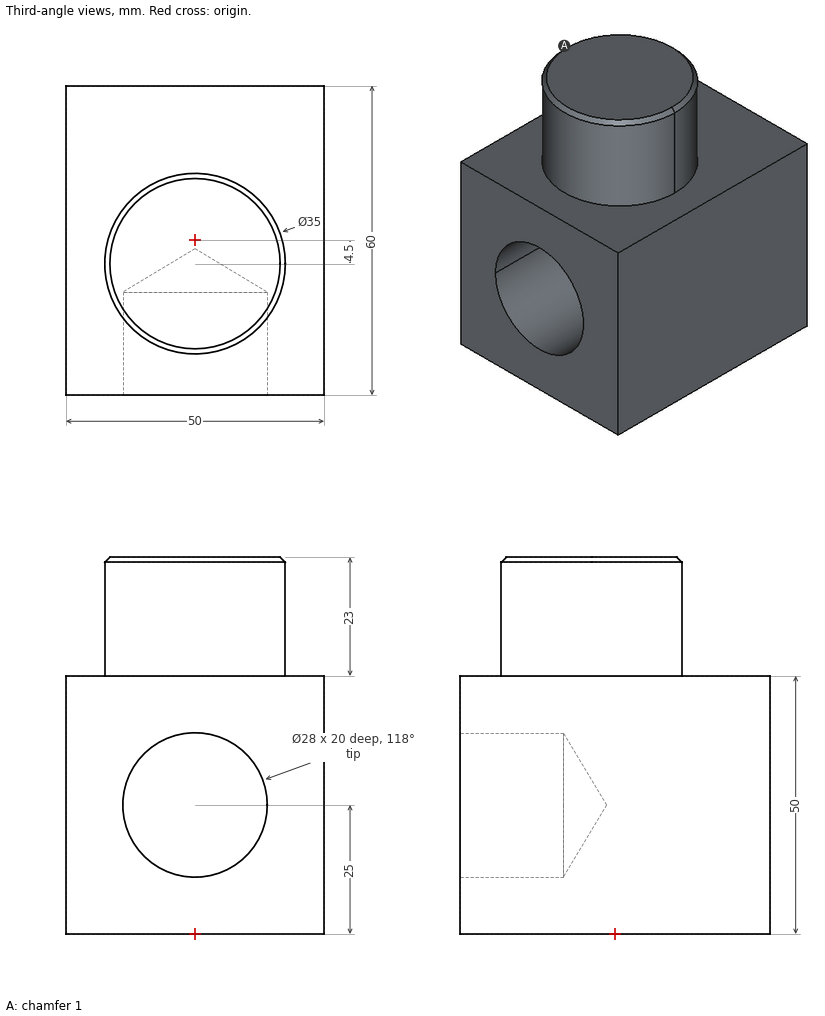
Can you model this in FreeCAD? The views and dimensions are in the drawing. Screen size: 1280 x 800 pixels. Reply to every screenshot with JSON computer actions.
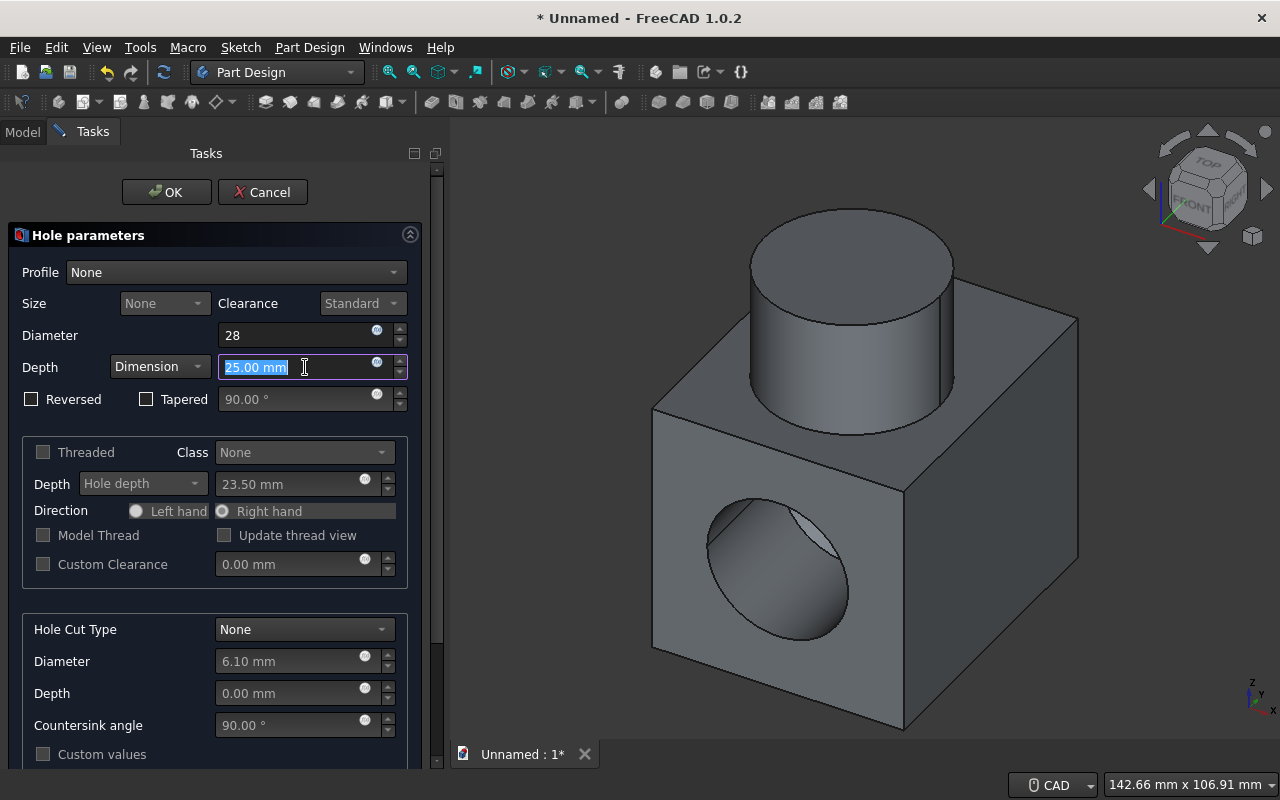
{"action": "type", "text": "20"}
{"action": "key", "text": "Tab"}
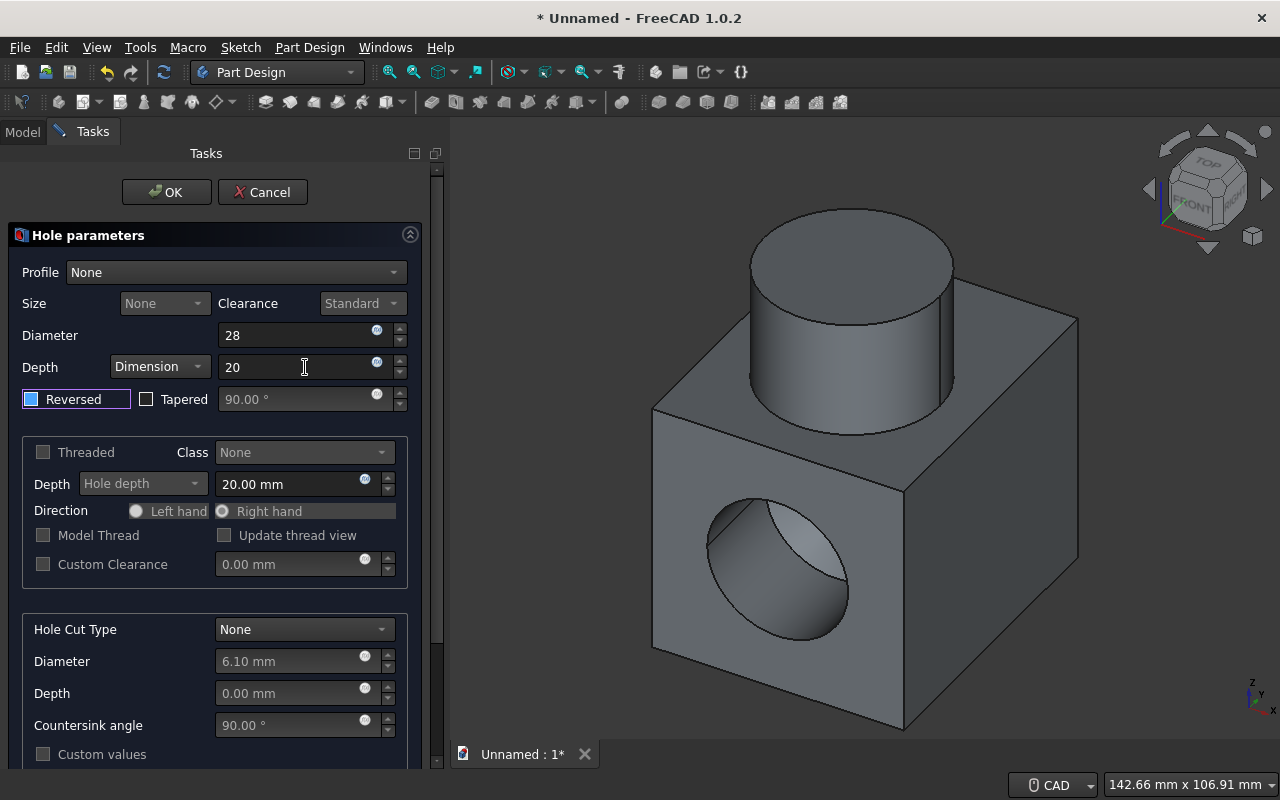
{"action": "left_click", "coordinate": [167, 192]}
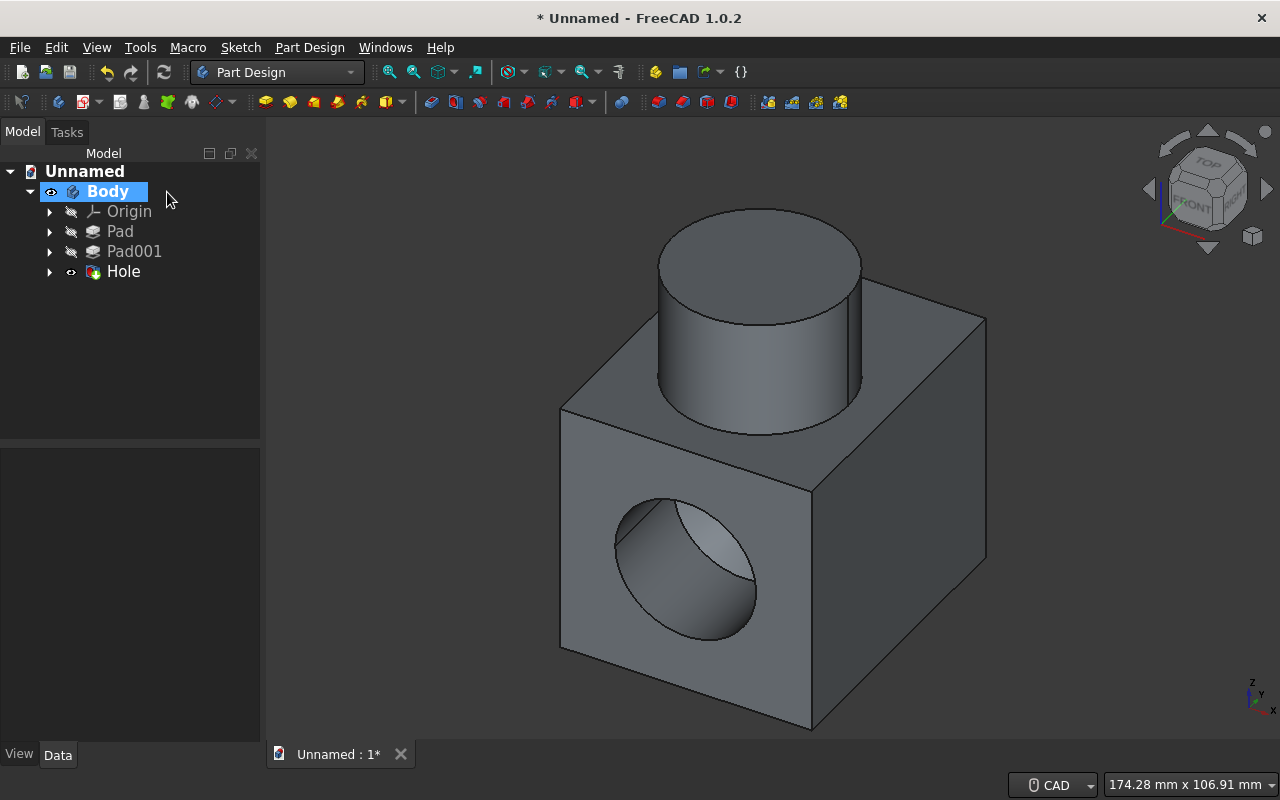
{"action": "left_click", "coordinate": [659, 272]}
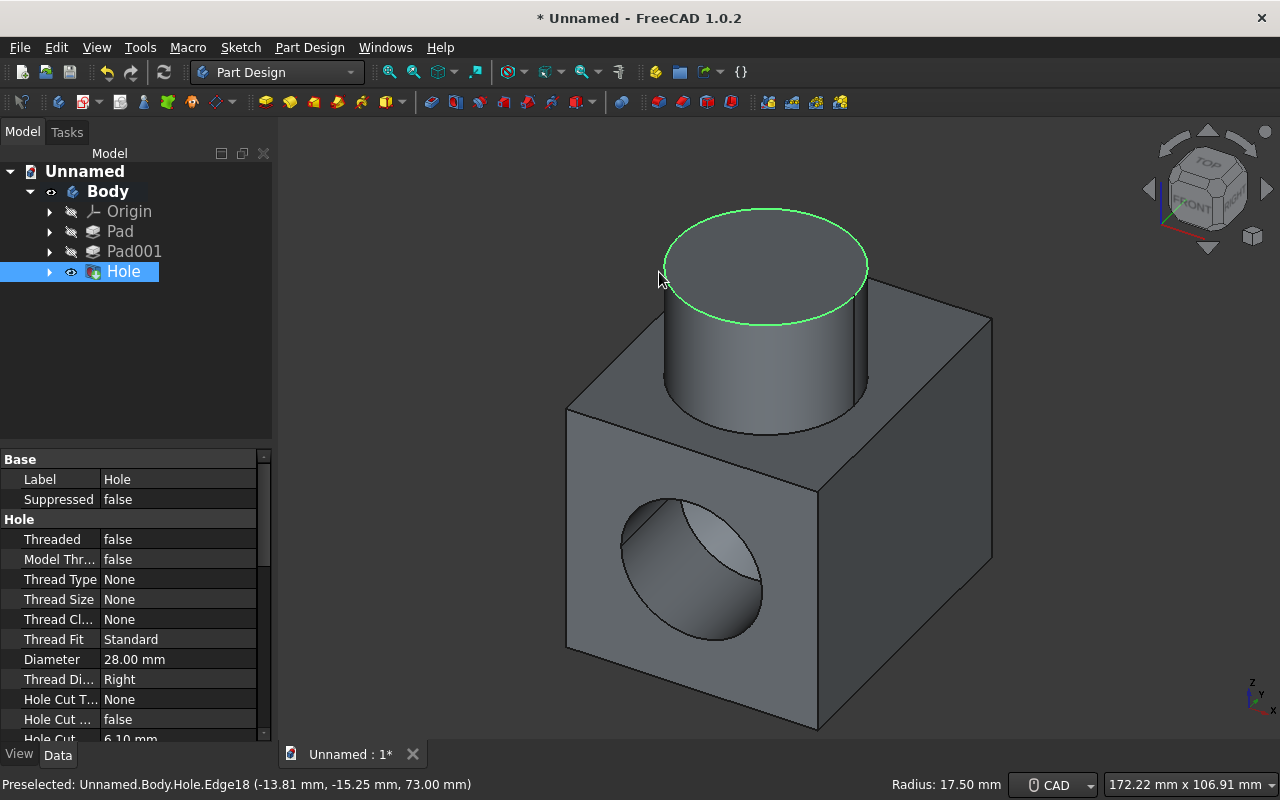
{"action": "left_click", "coordinate": [684, 102]}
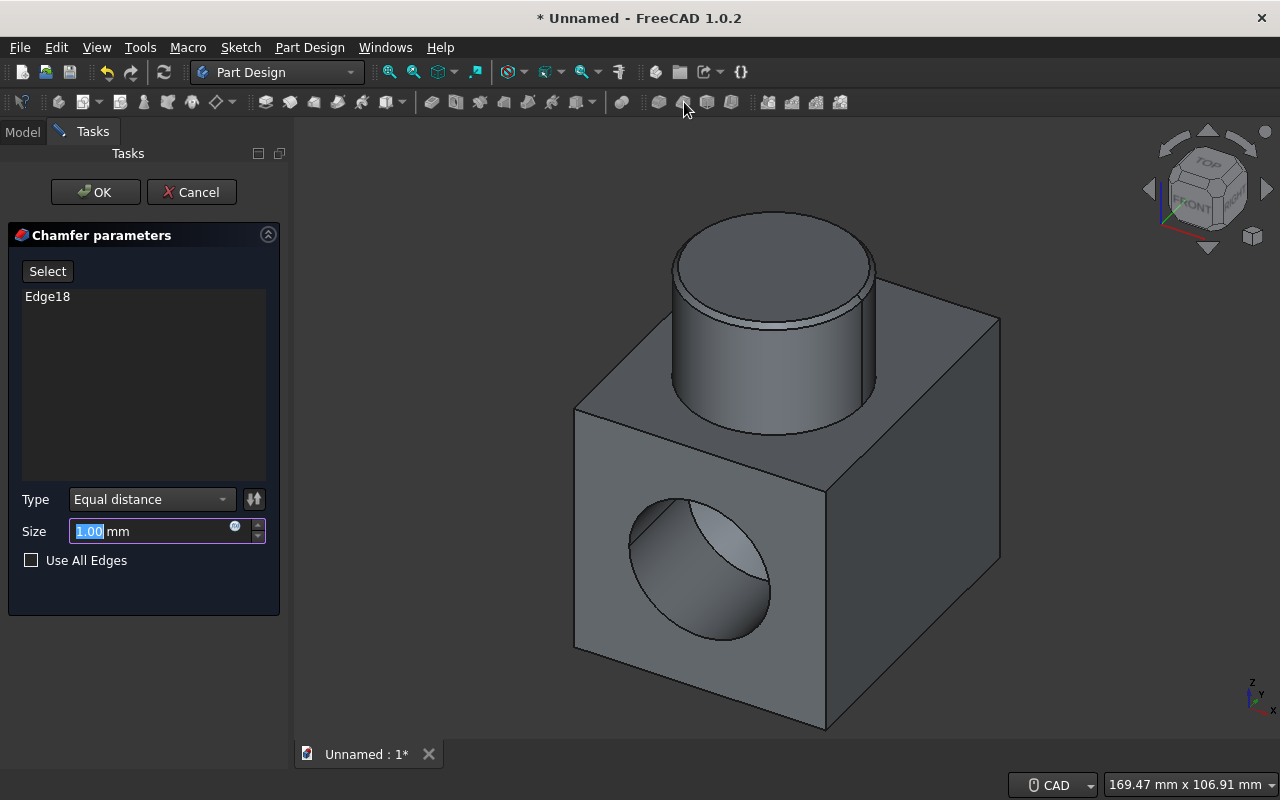
{"action": "type", "text": "1"}
{"action": "key", "text": "Tab"}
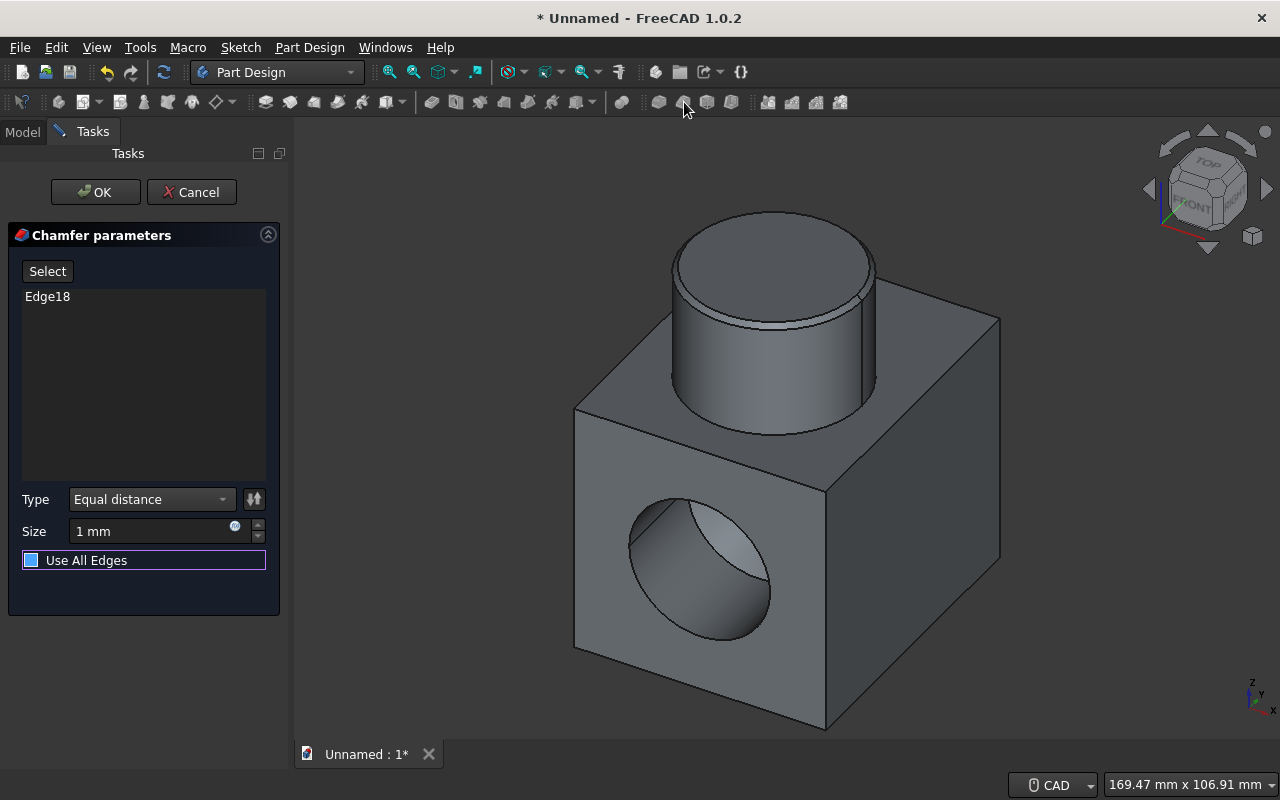
{"action": "left_click", "coordinate": [96, 192]}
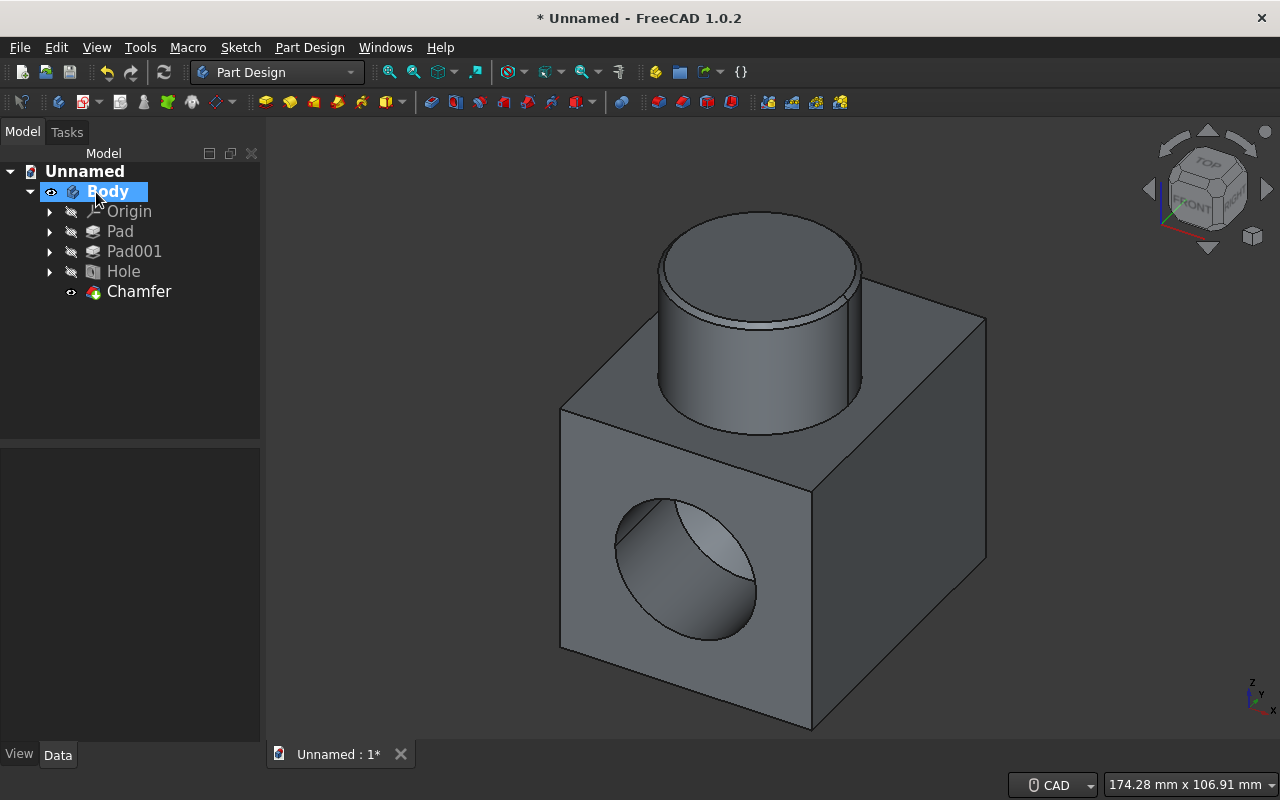
{"action": "key", "text": "0"}